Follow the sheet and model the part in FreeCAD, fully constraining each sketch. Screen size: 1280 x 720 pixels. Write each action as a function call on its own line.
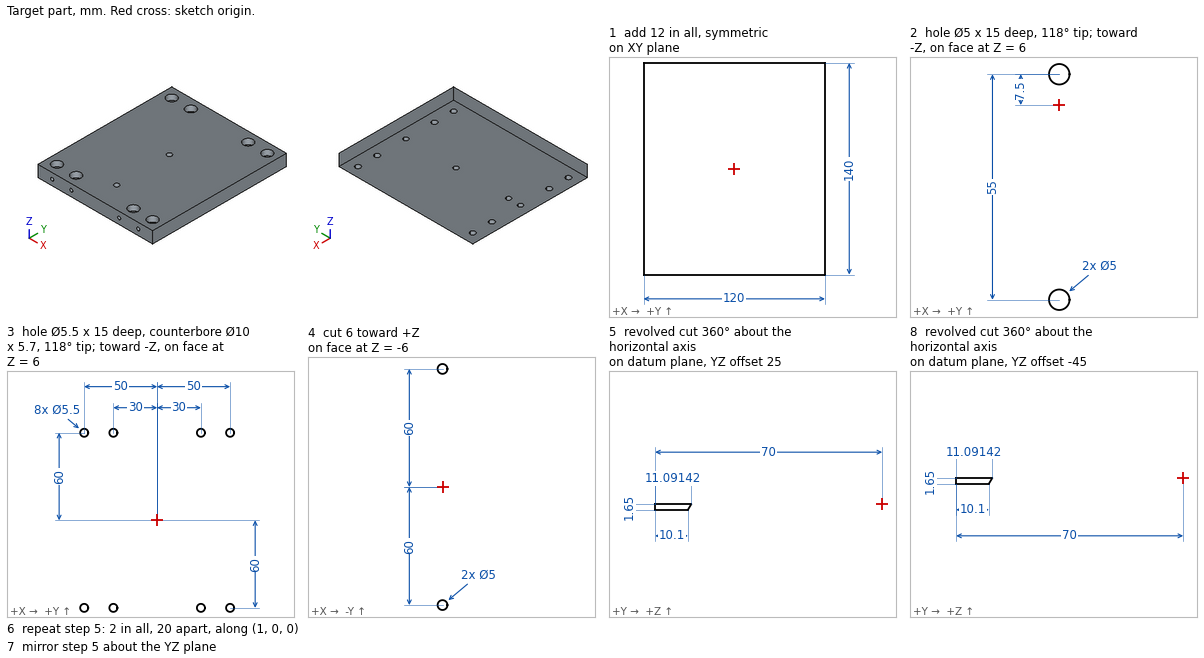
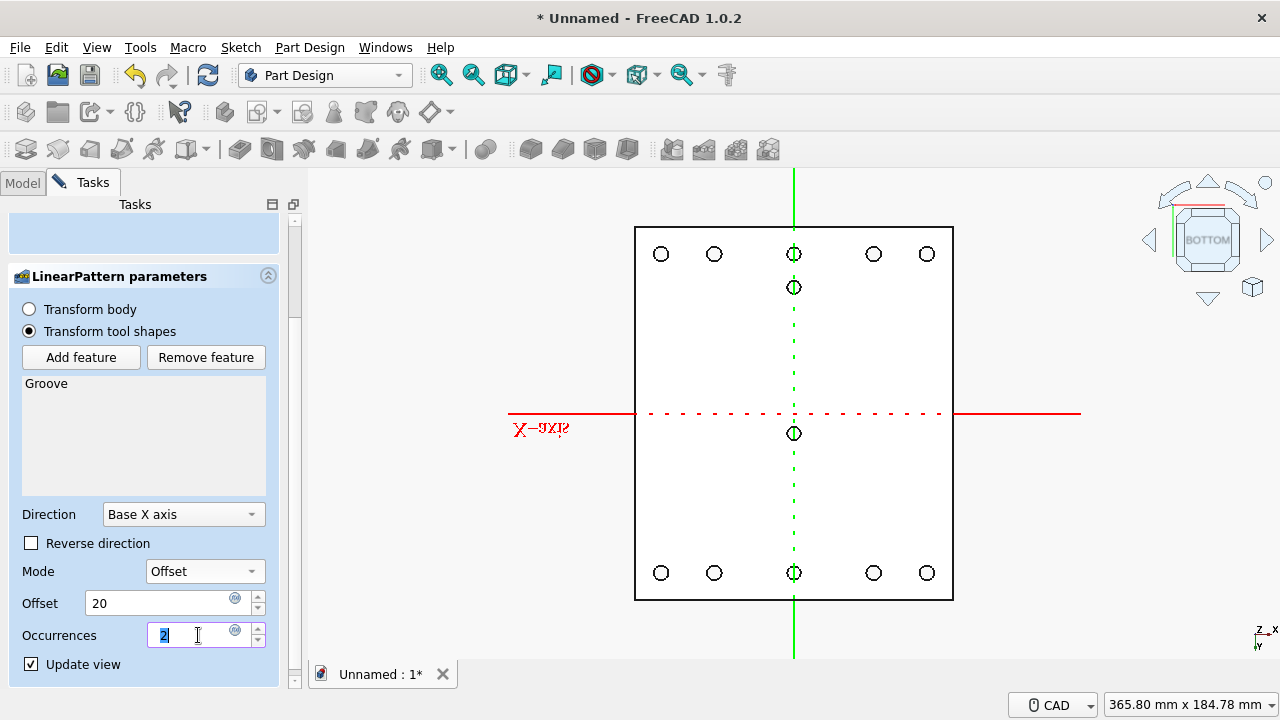
text(2)
key(Tab)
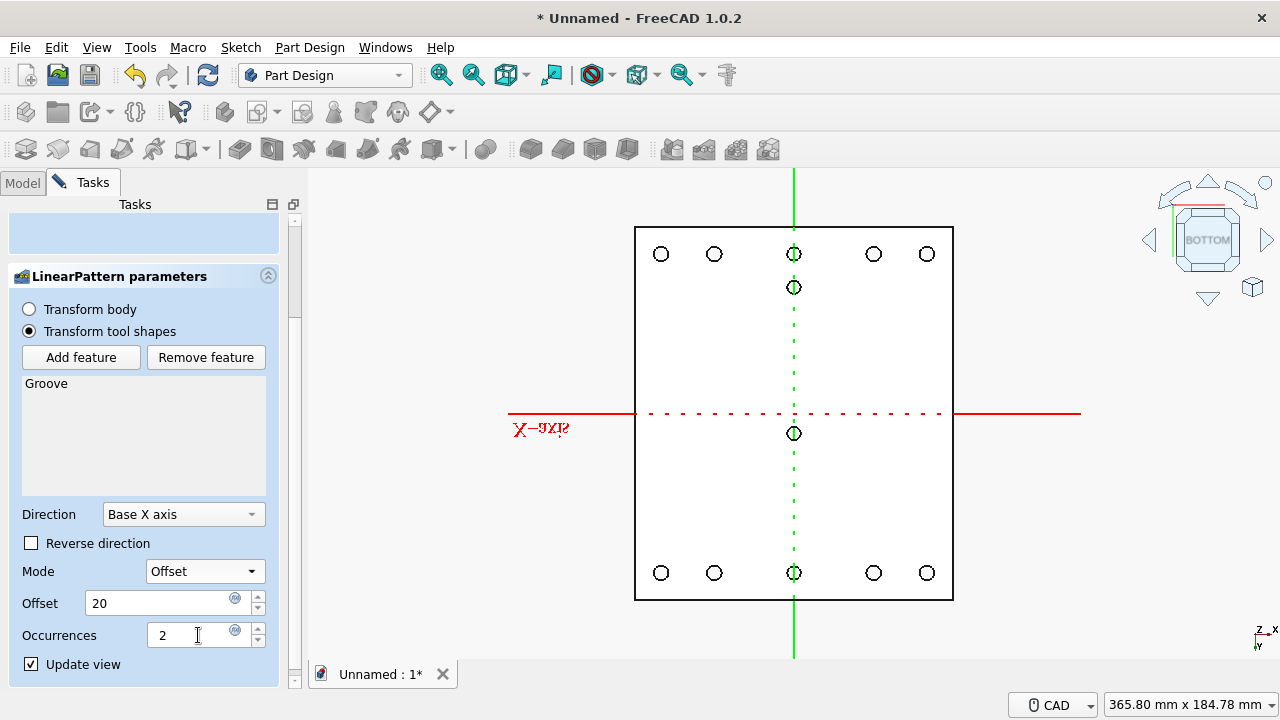
scroll(295, 451, up, 3)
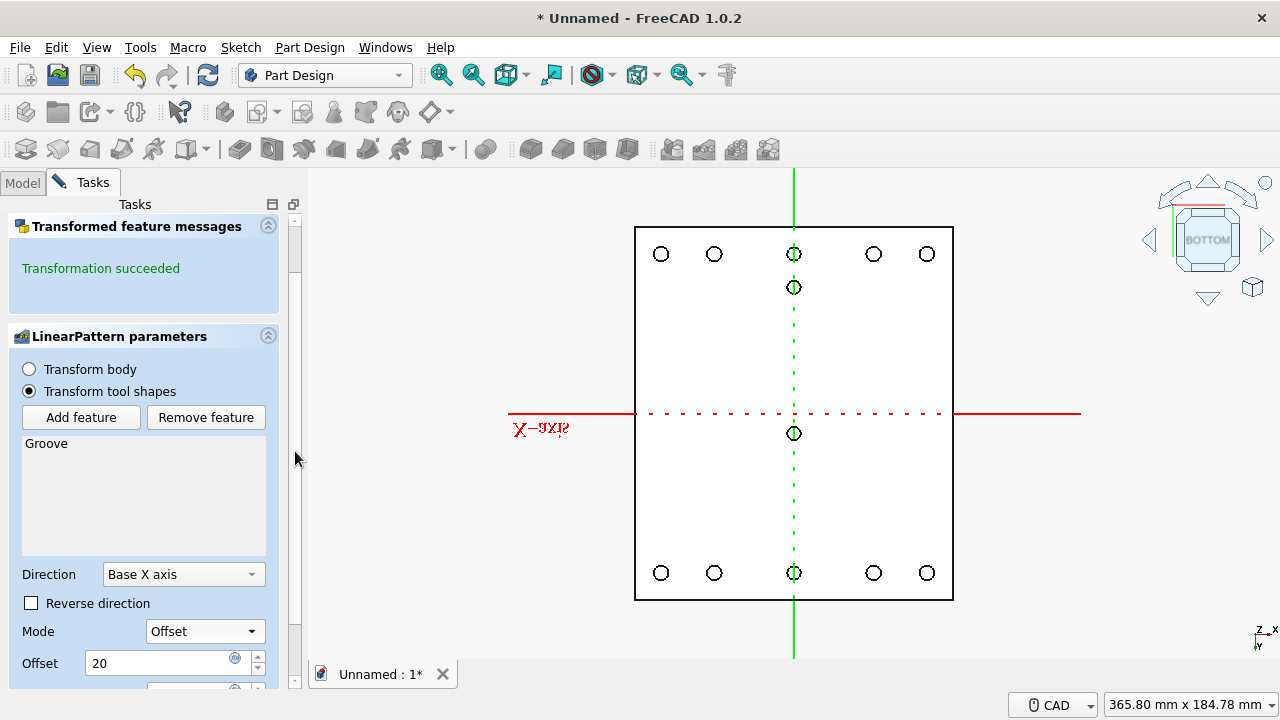
click(96, 243)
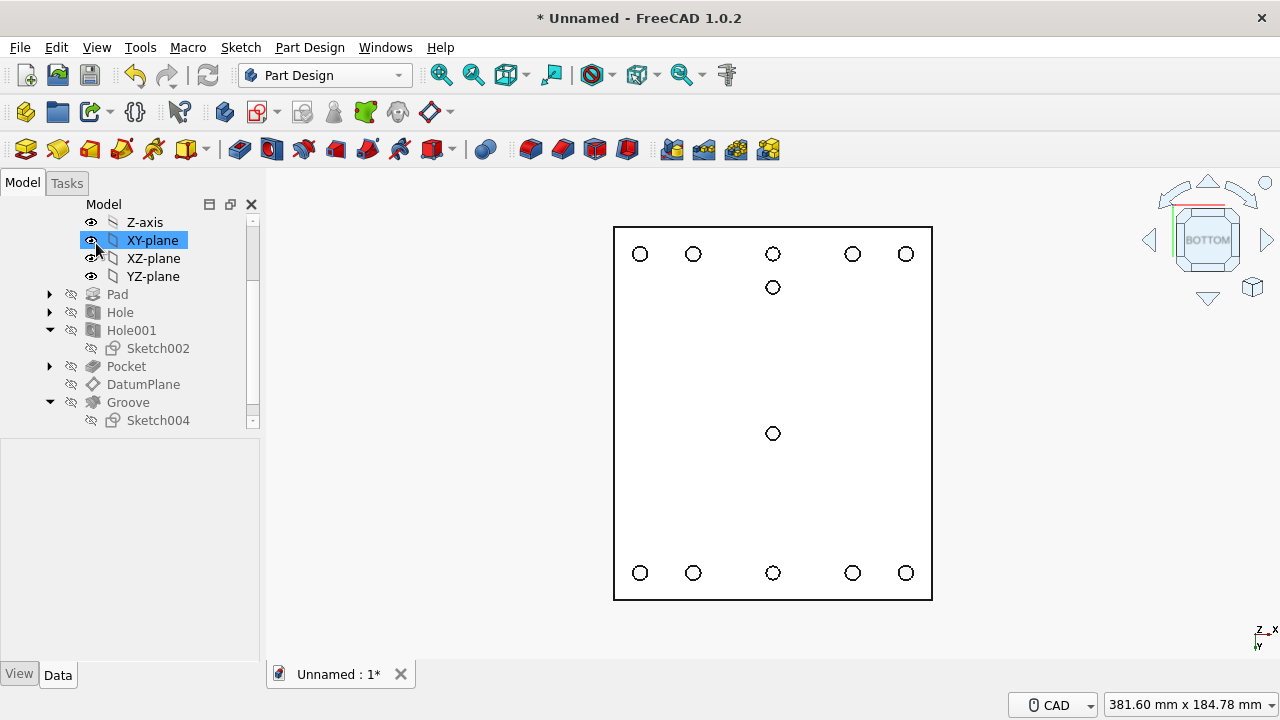
click(116, 402)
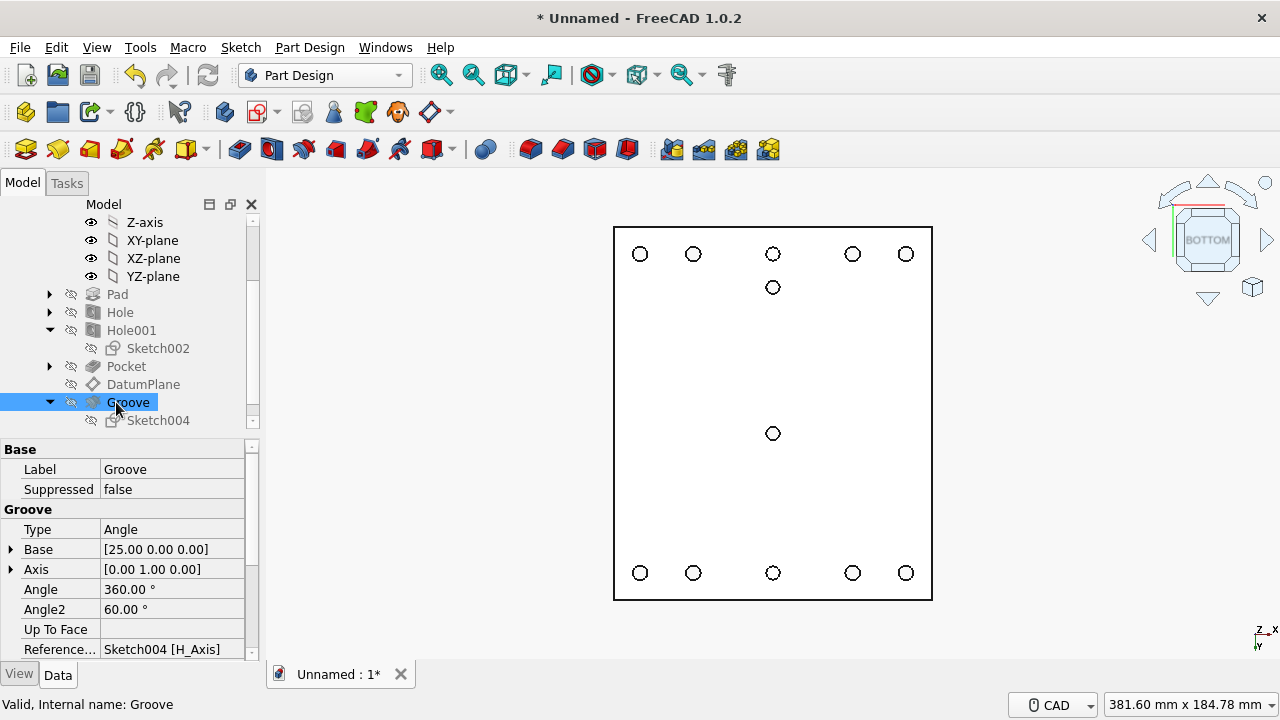
click(672, 150)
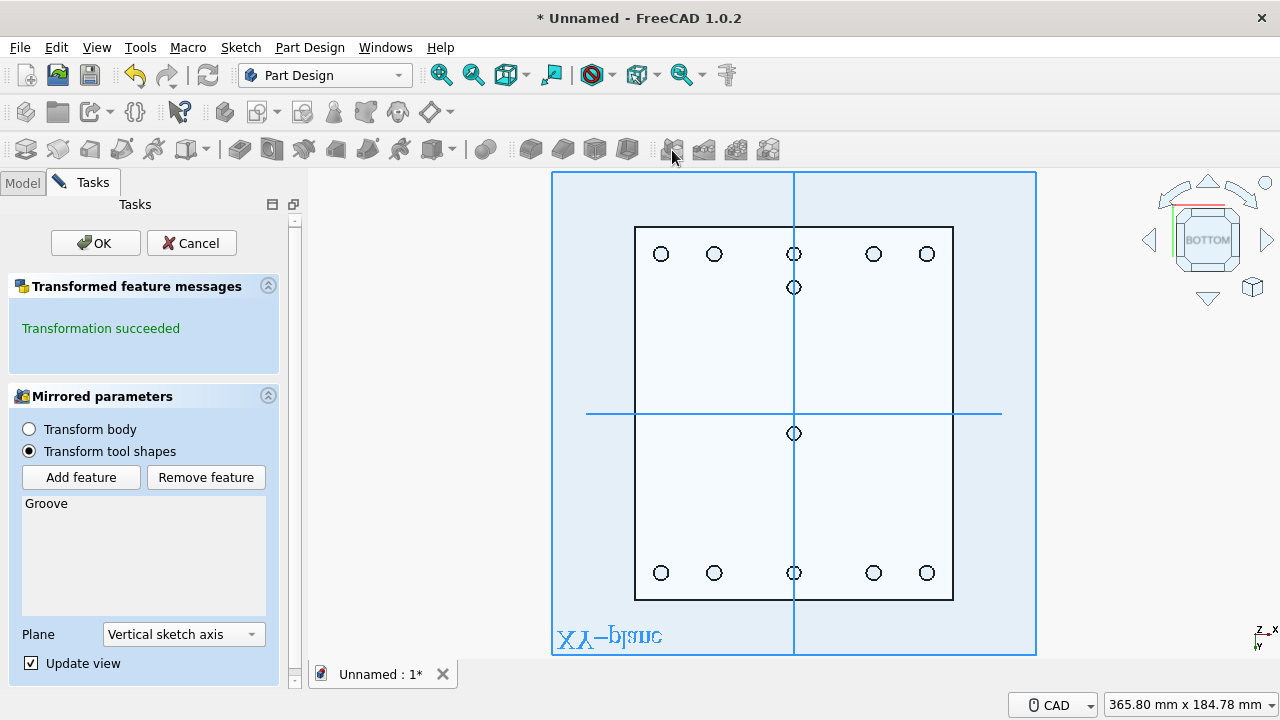
click(184, 634)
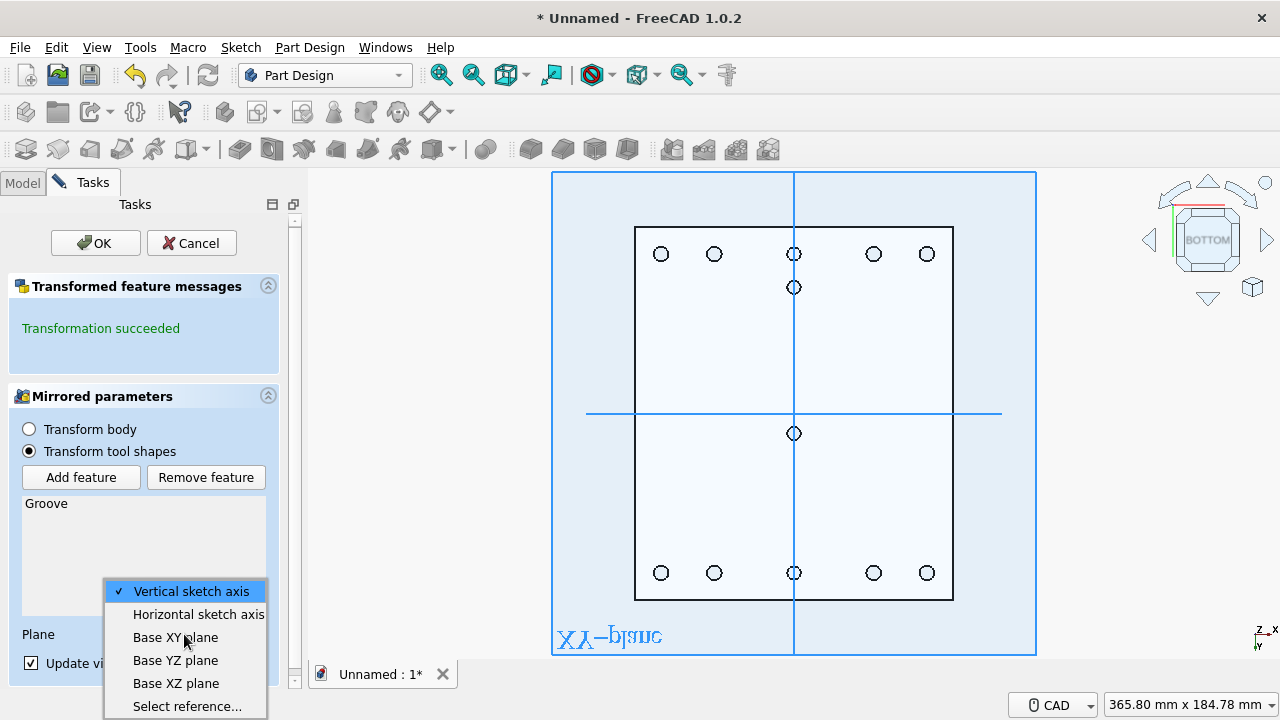
click(184, 660)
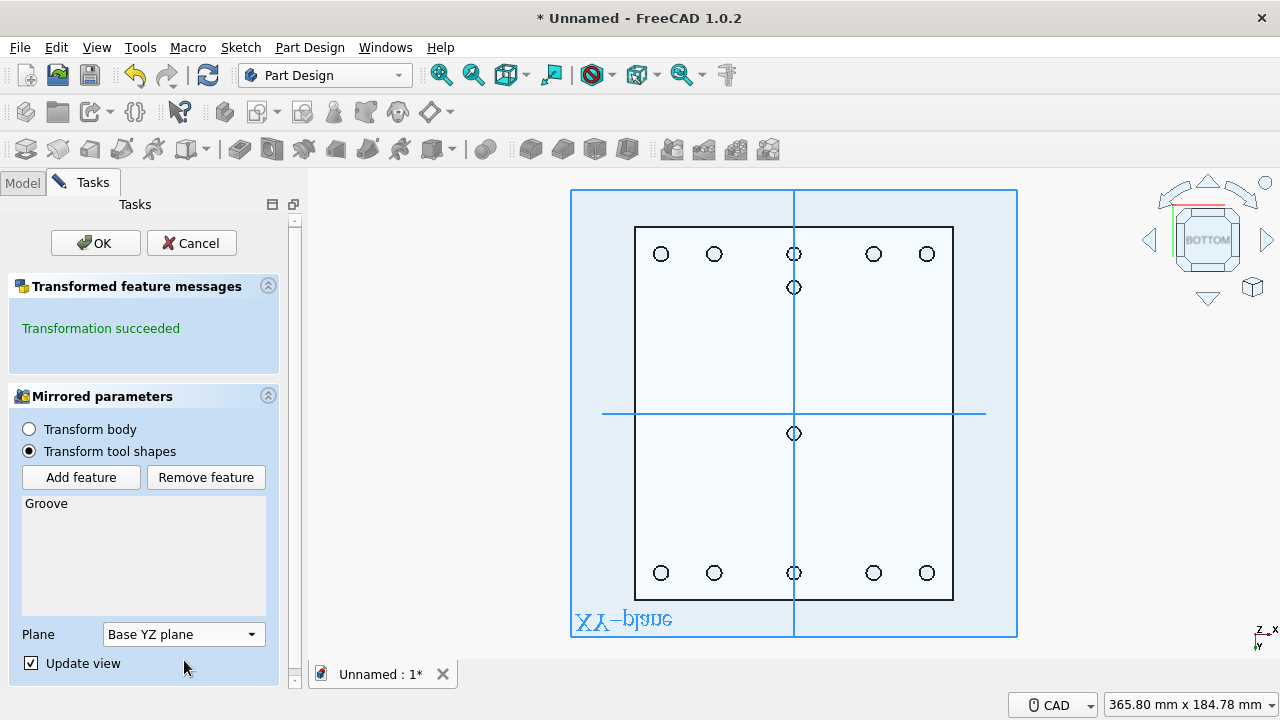
click(96, 243)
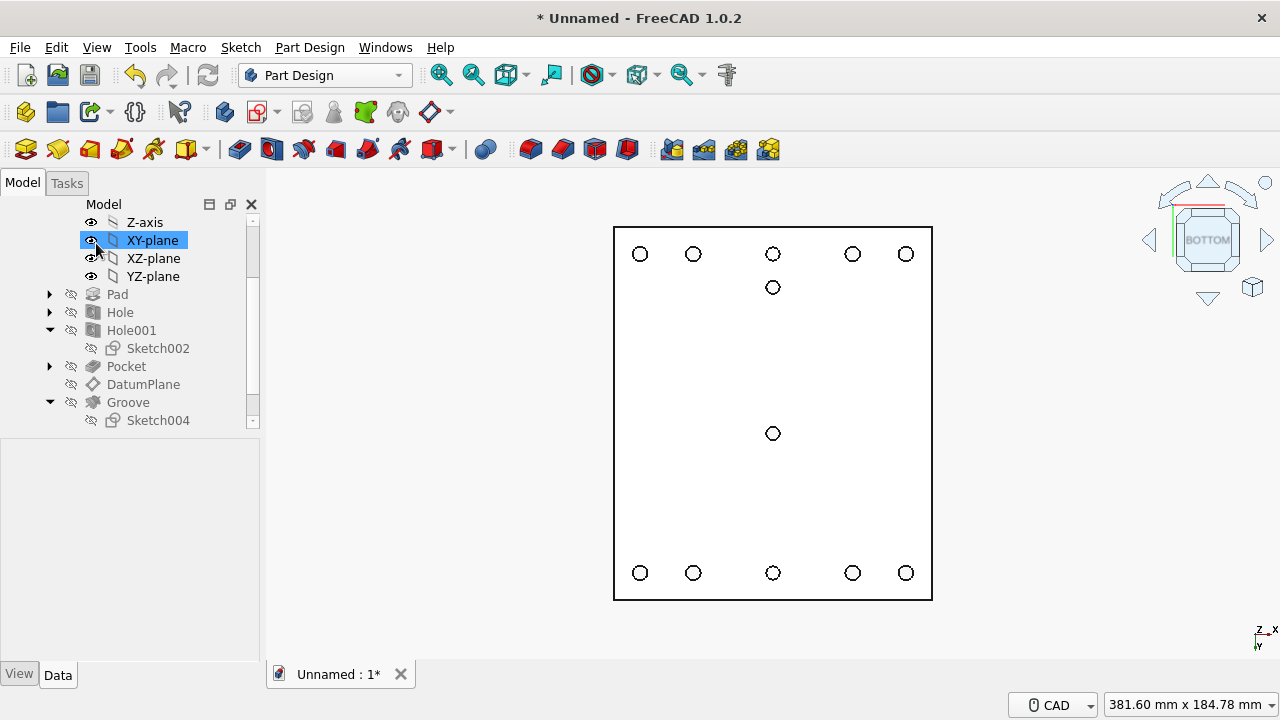
scroll(160, 326, down, 3)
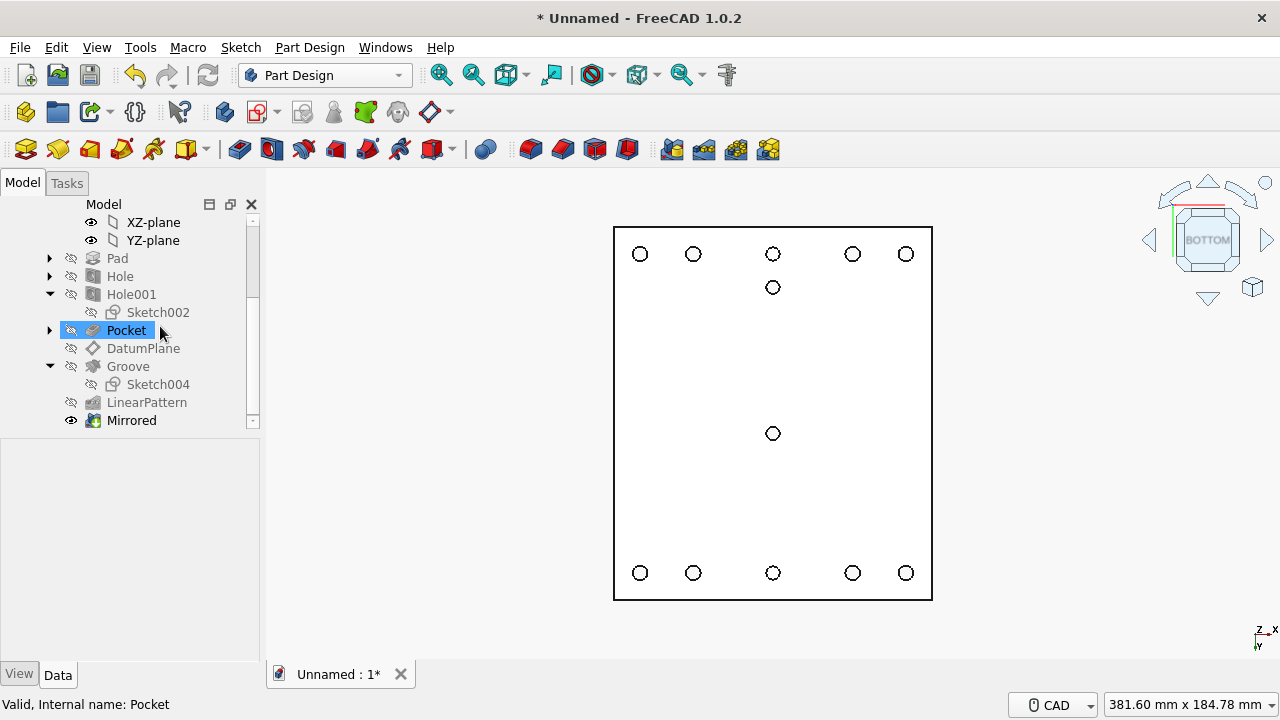
scroll(160, 326, up, 15)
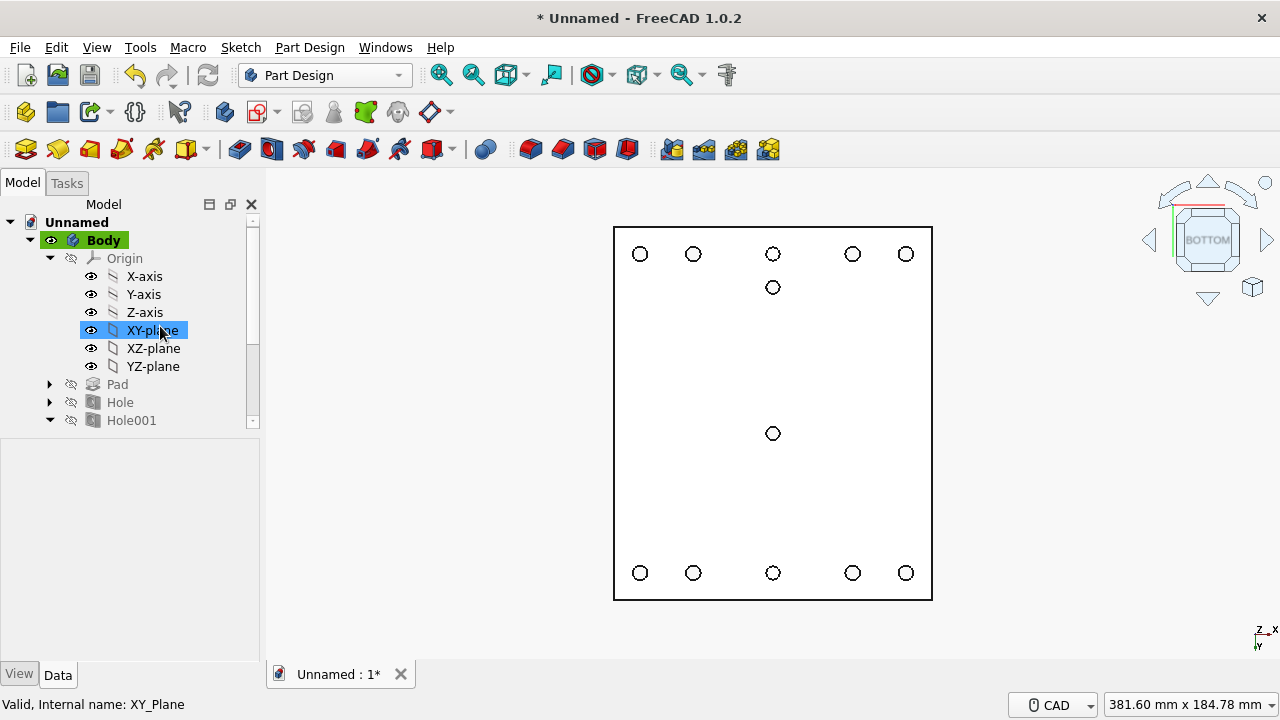
click(136, 366)